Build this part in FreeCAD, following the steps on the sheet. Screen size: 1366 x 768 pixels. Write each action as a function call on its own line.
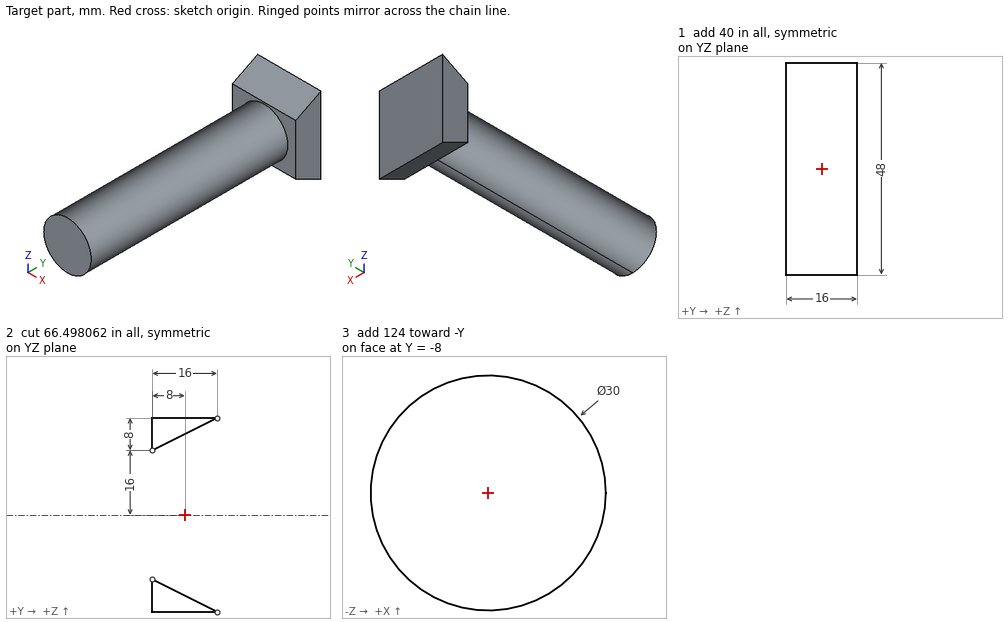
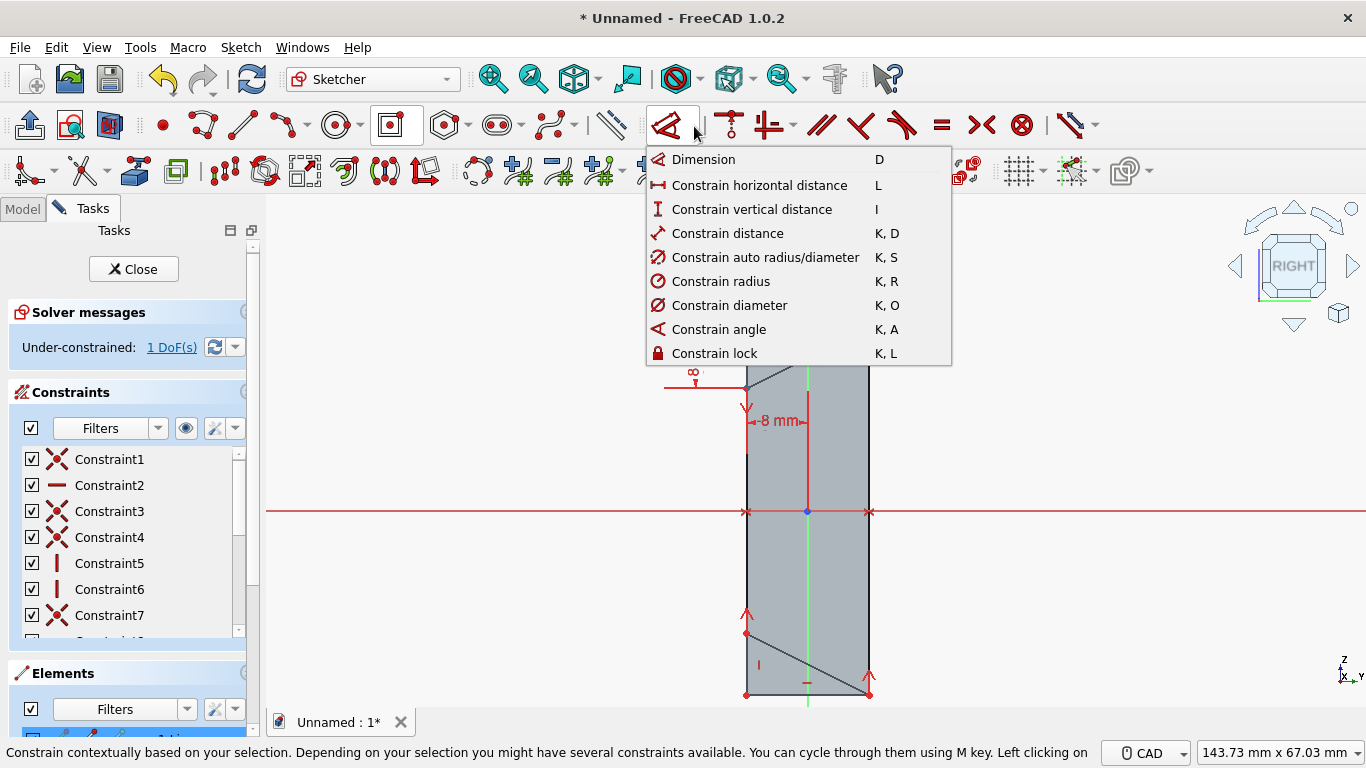
click(799, 209)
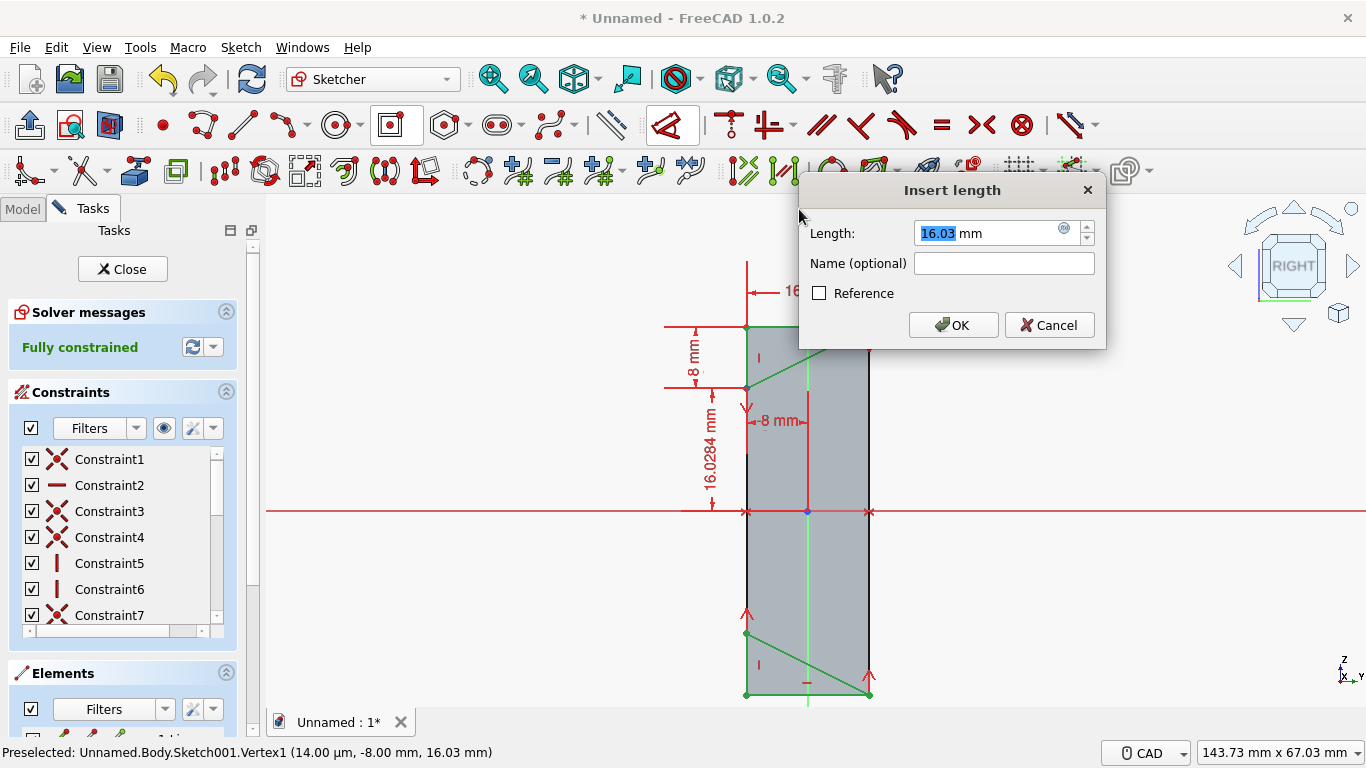
text(16)
key(Return)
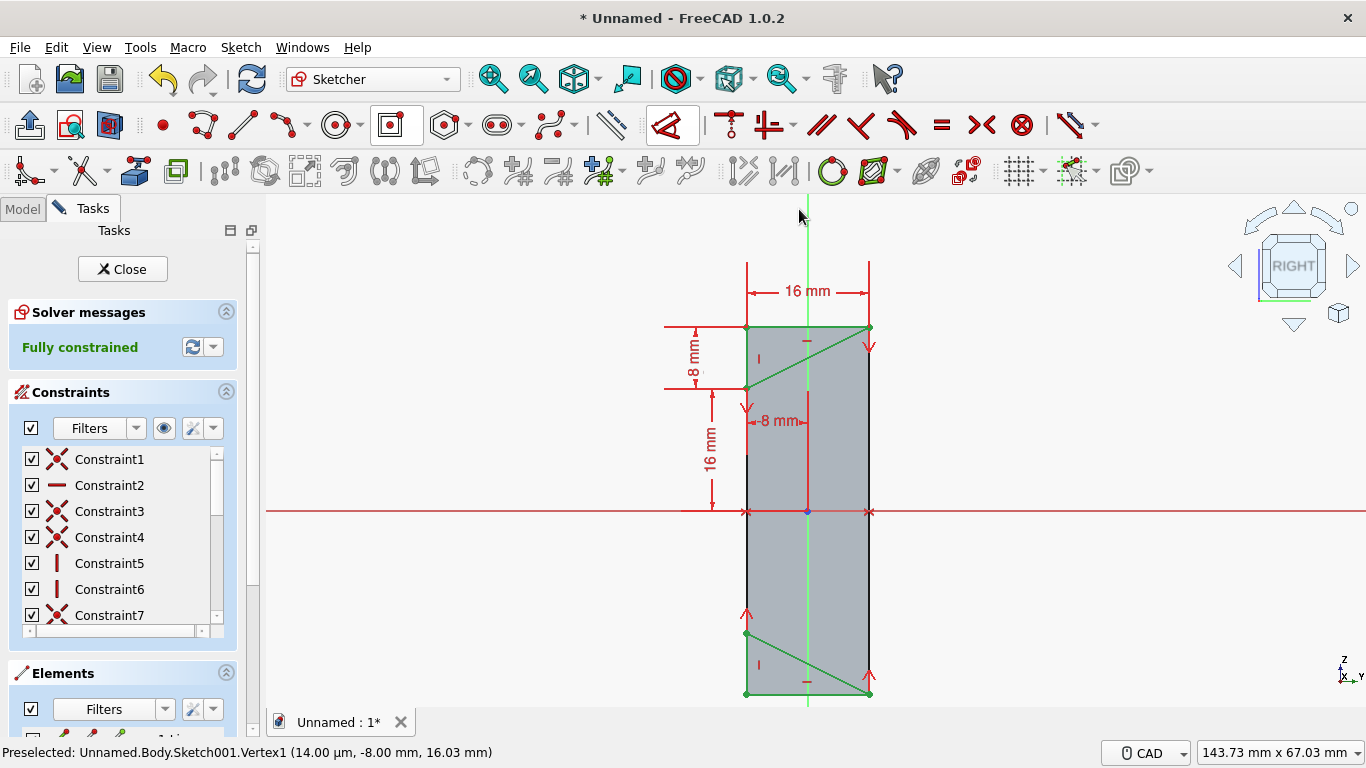
click(123, 269)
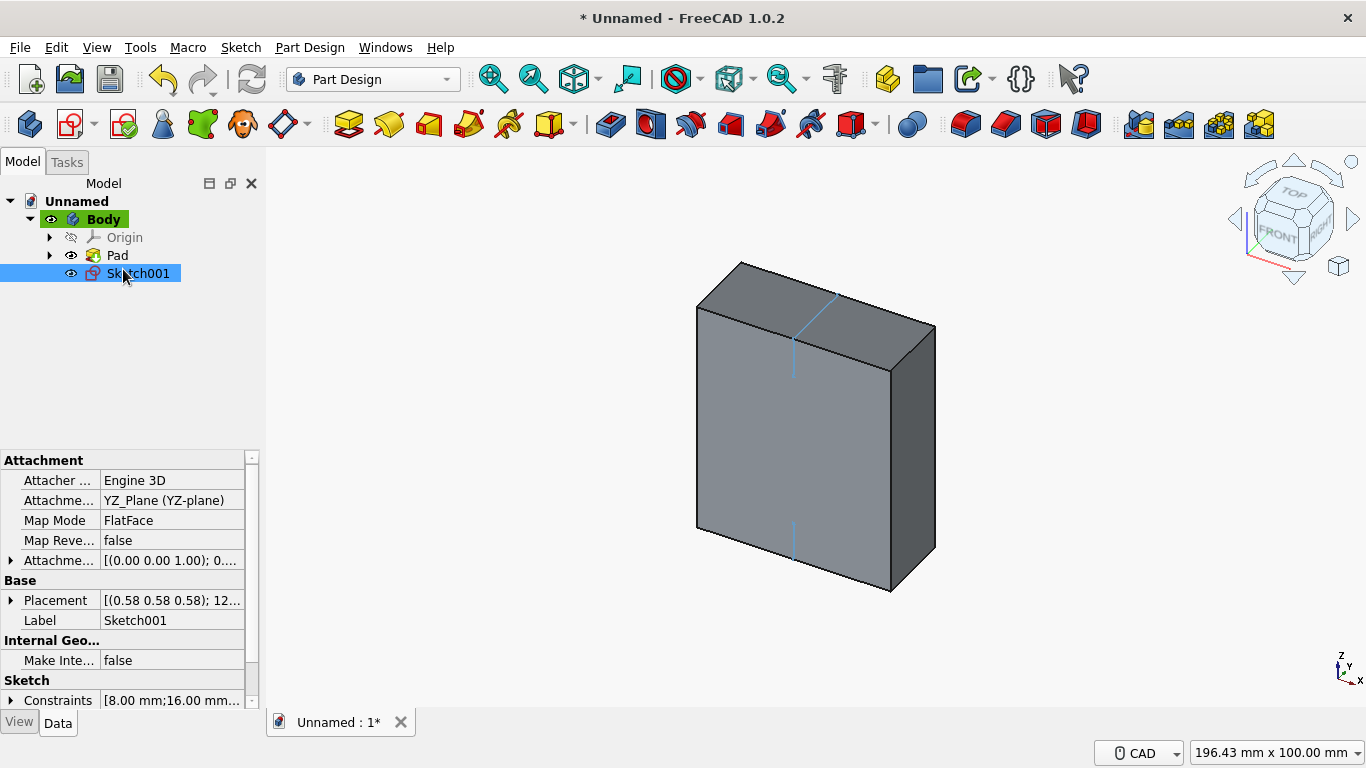
click(612, 124)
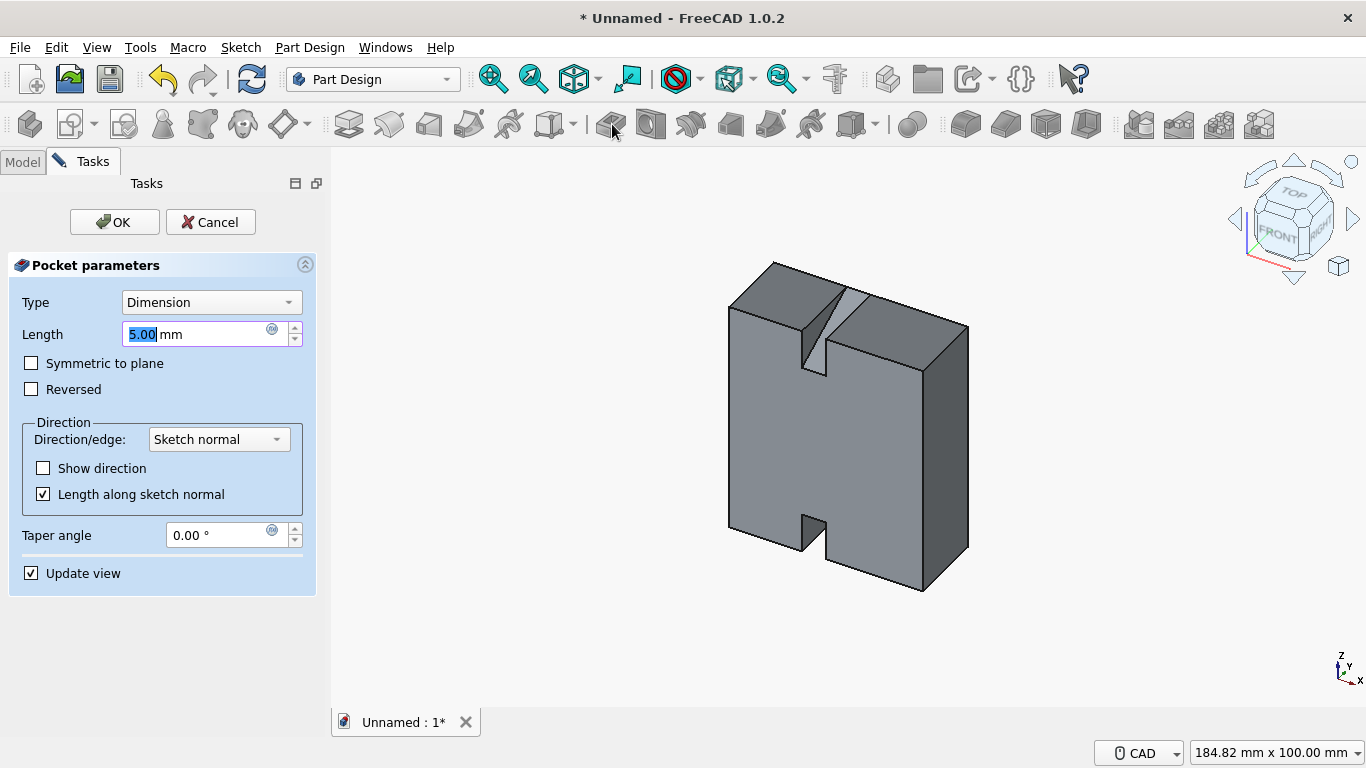
text(66.498062)
key(Tab)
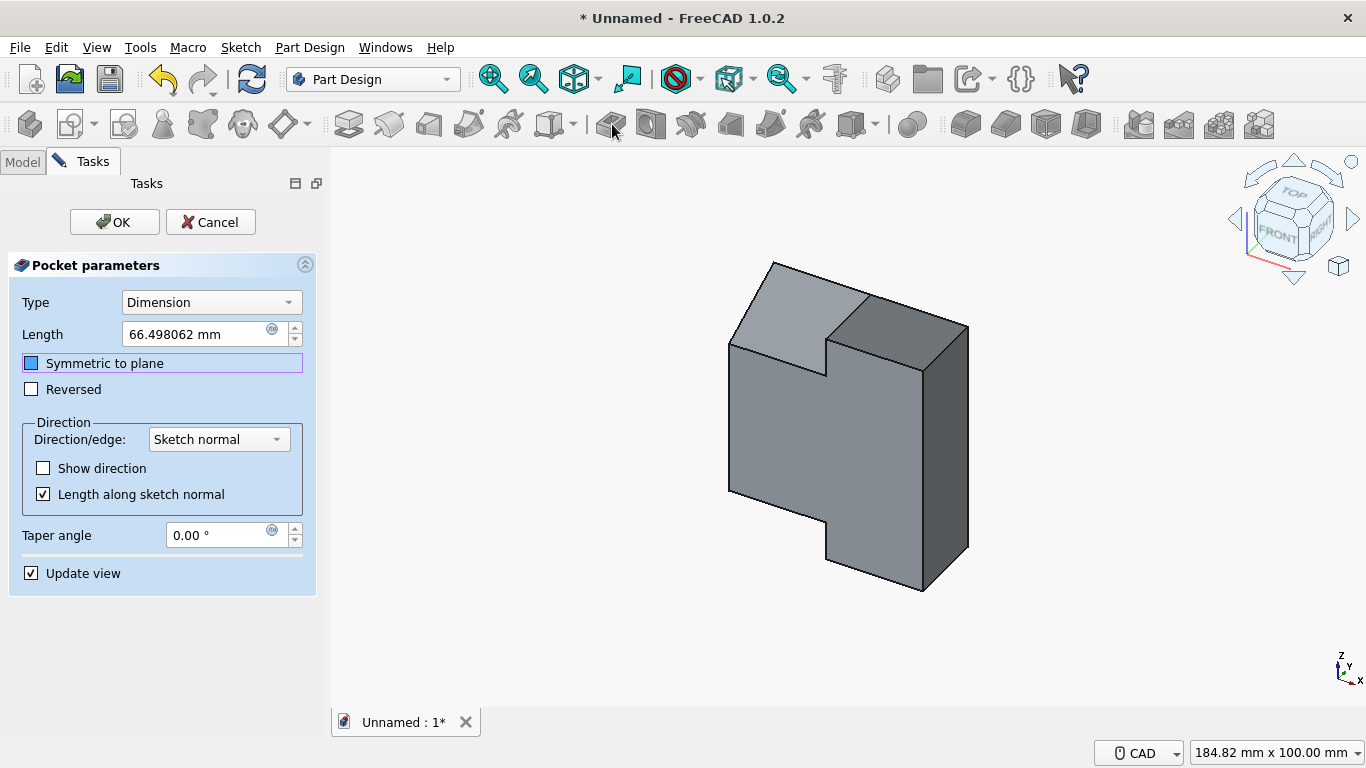
click(30, 363)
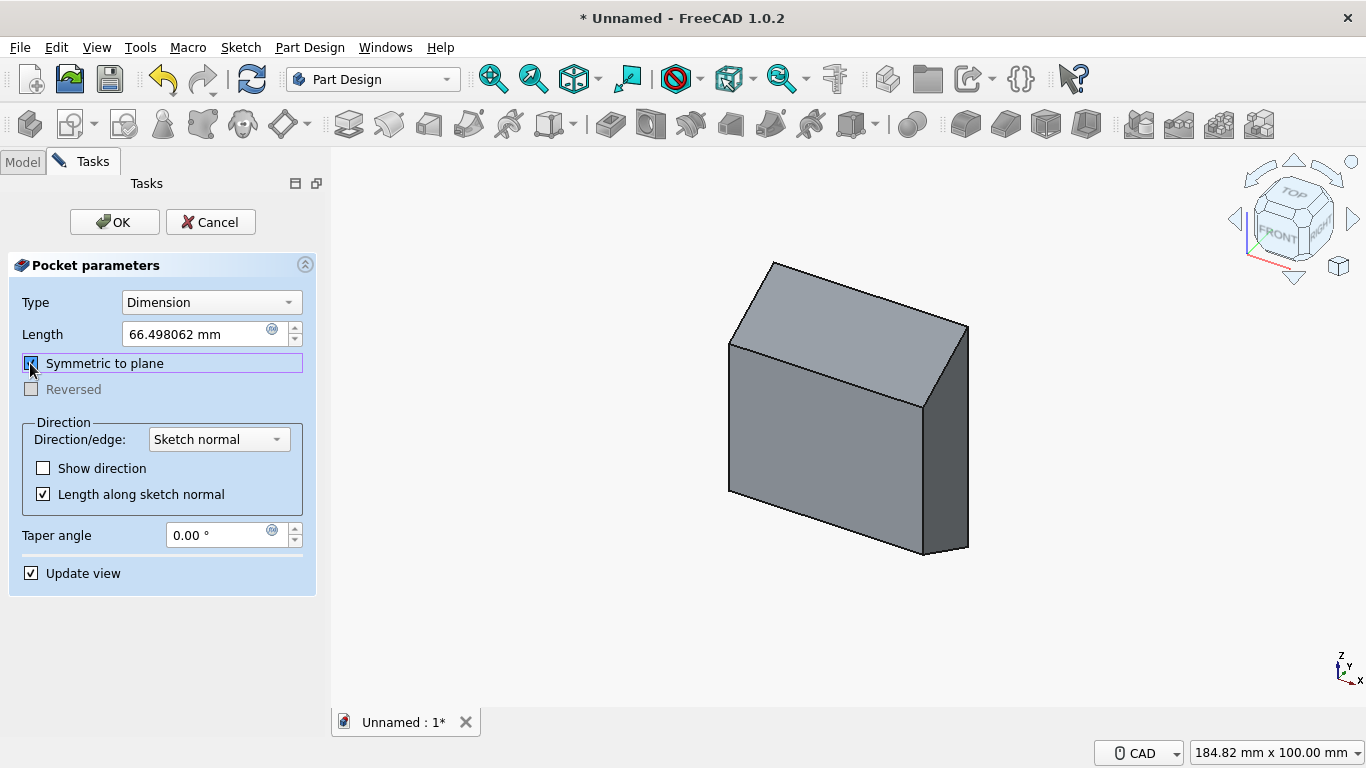
click(115, 222)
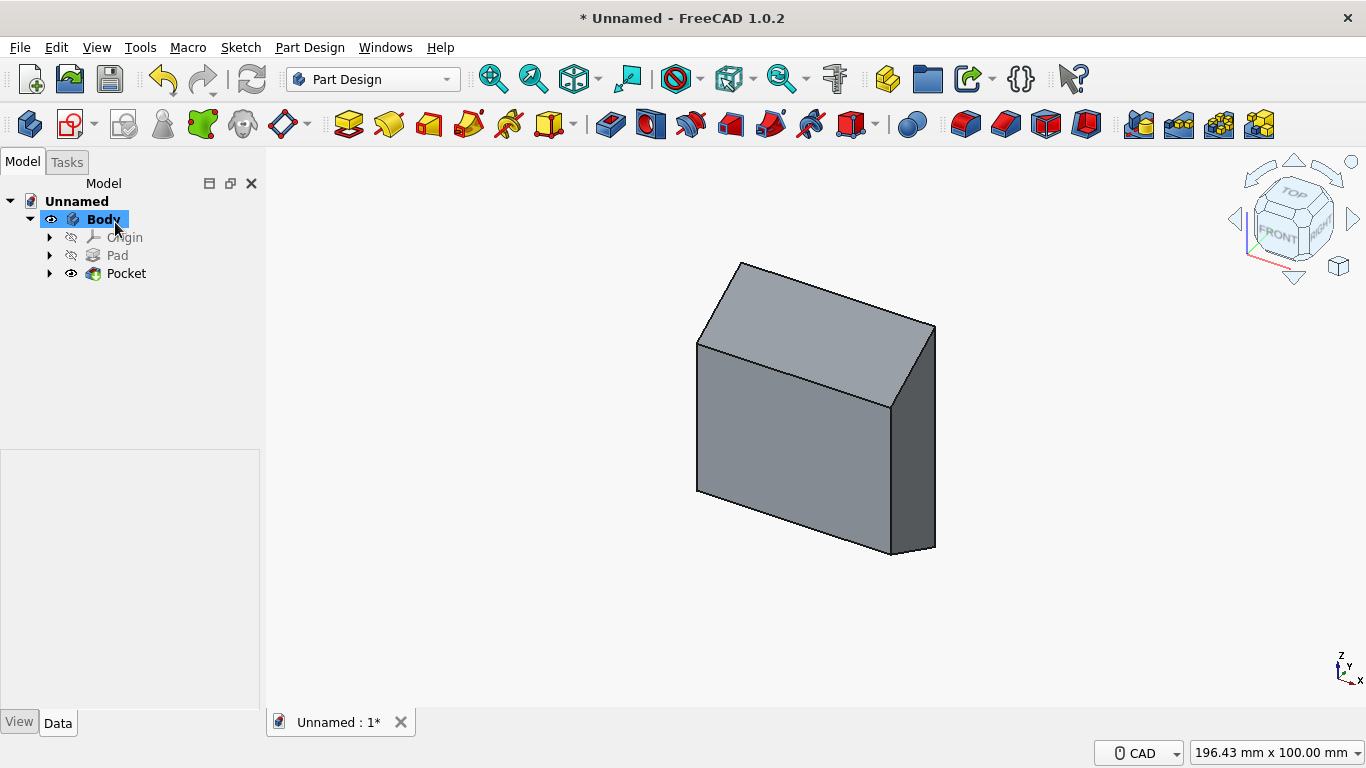
click(794, 448)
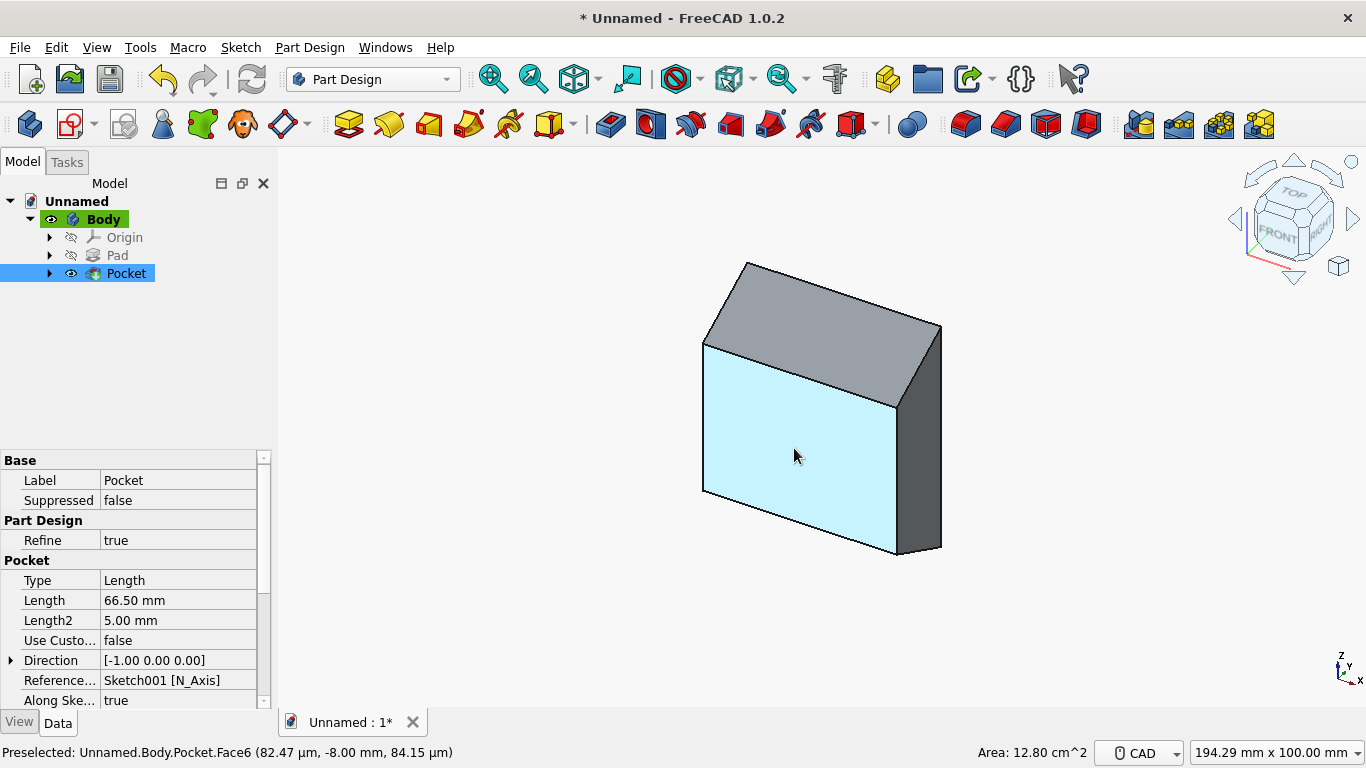
click(70, 124)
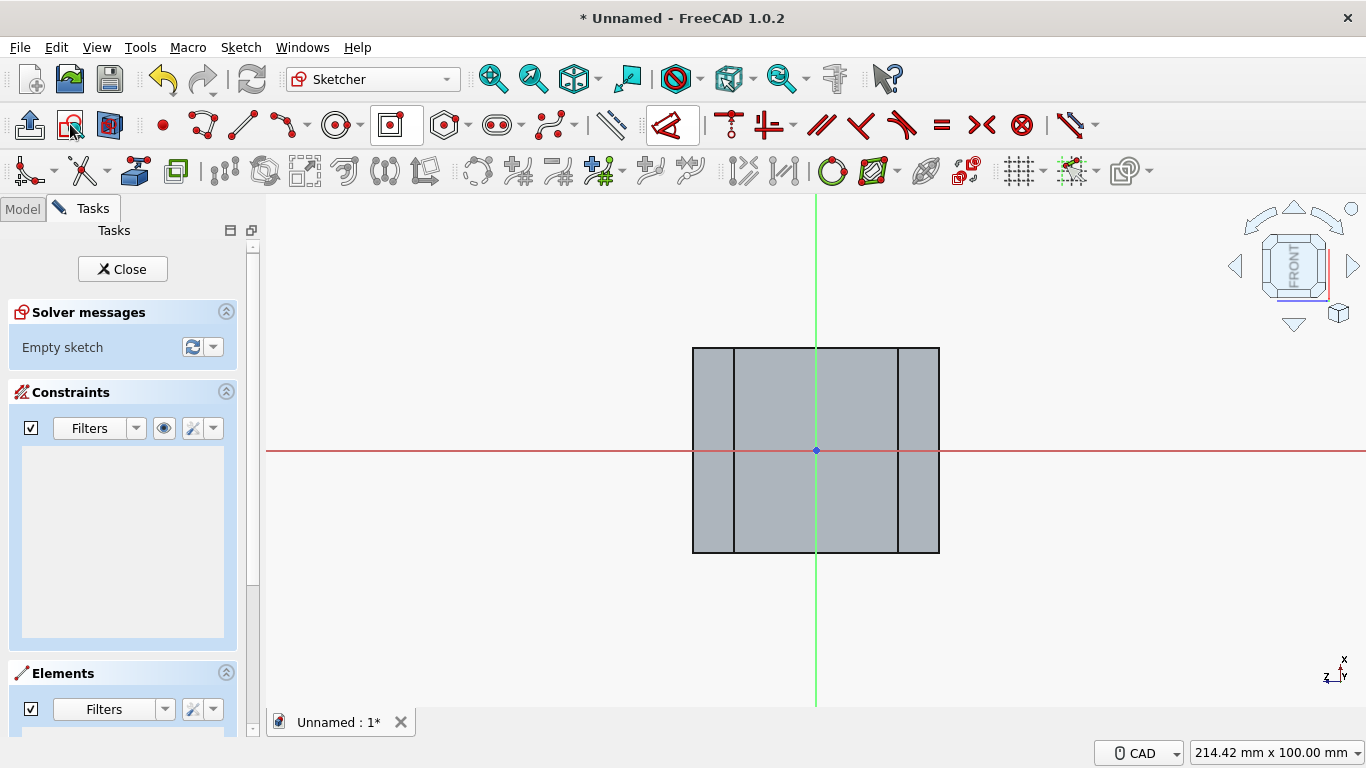
scroll(872, 451, up, 4)